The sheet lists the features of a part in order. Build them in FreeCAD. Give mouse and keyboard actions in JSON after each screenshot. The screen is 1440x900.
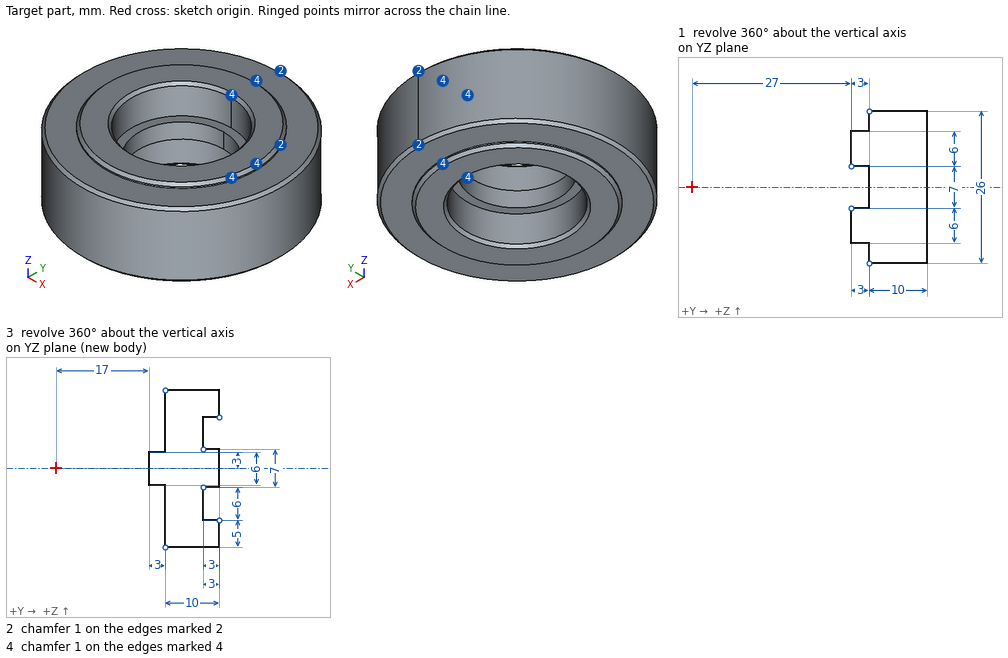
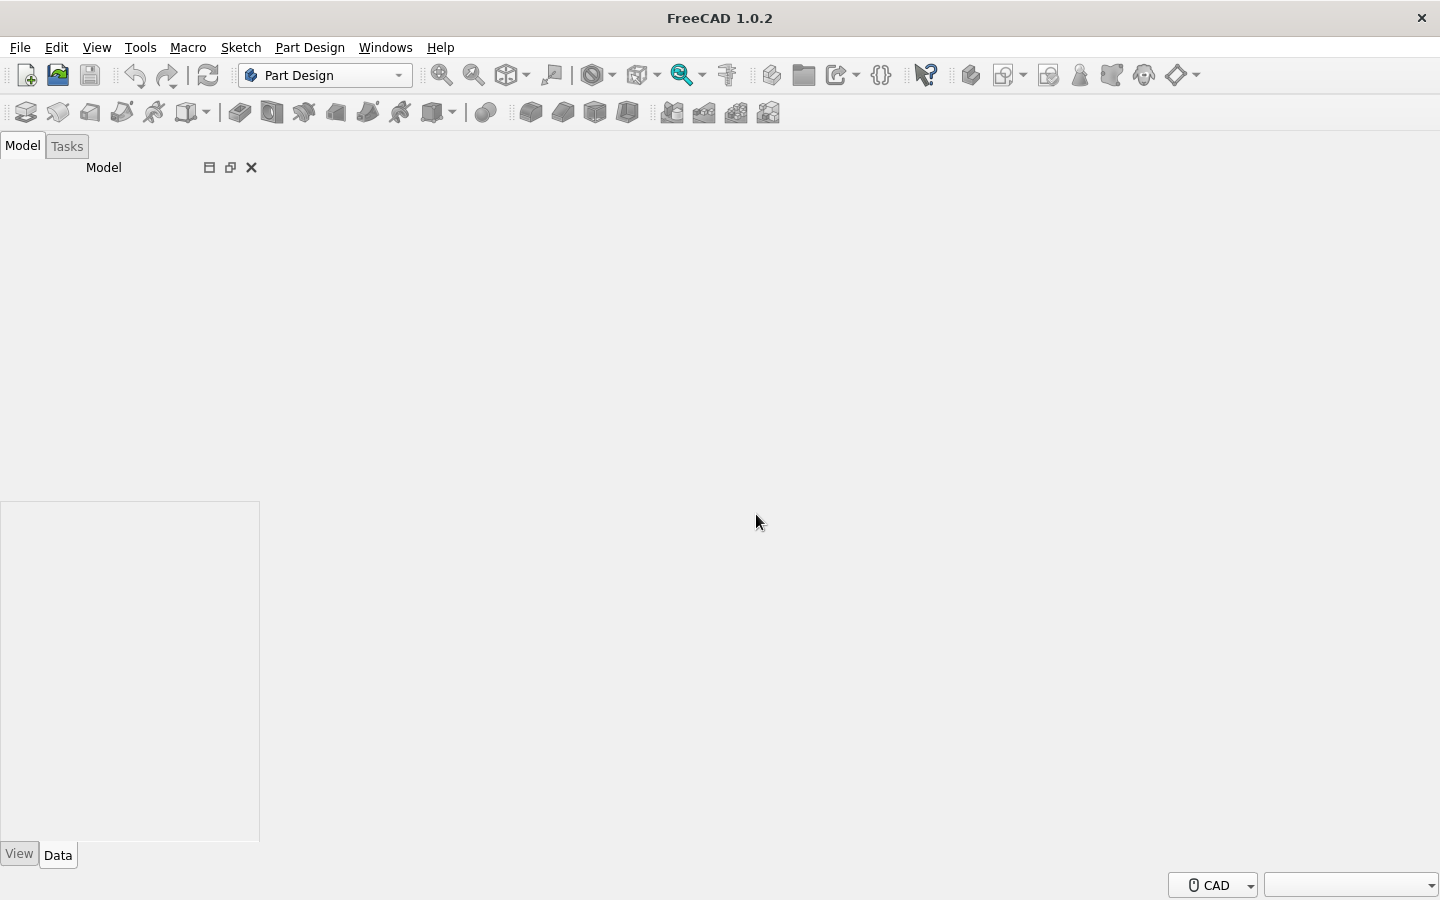
{"action": "left_click", "coordinate": [26, 76]}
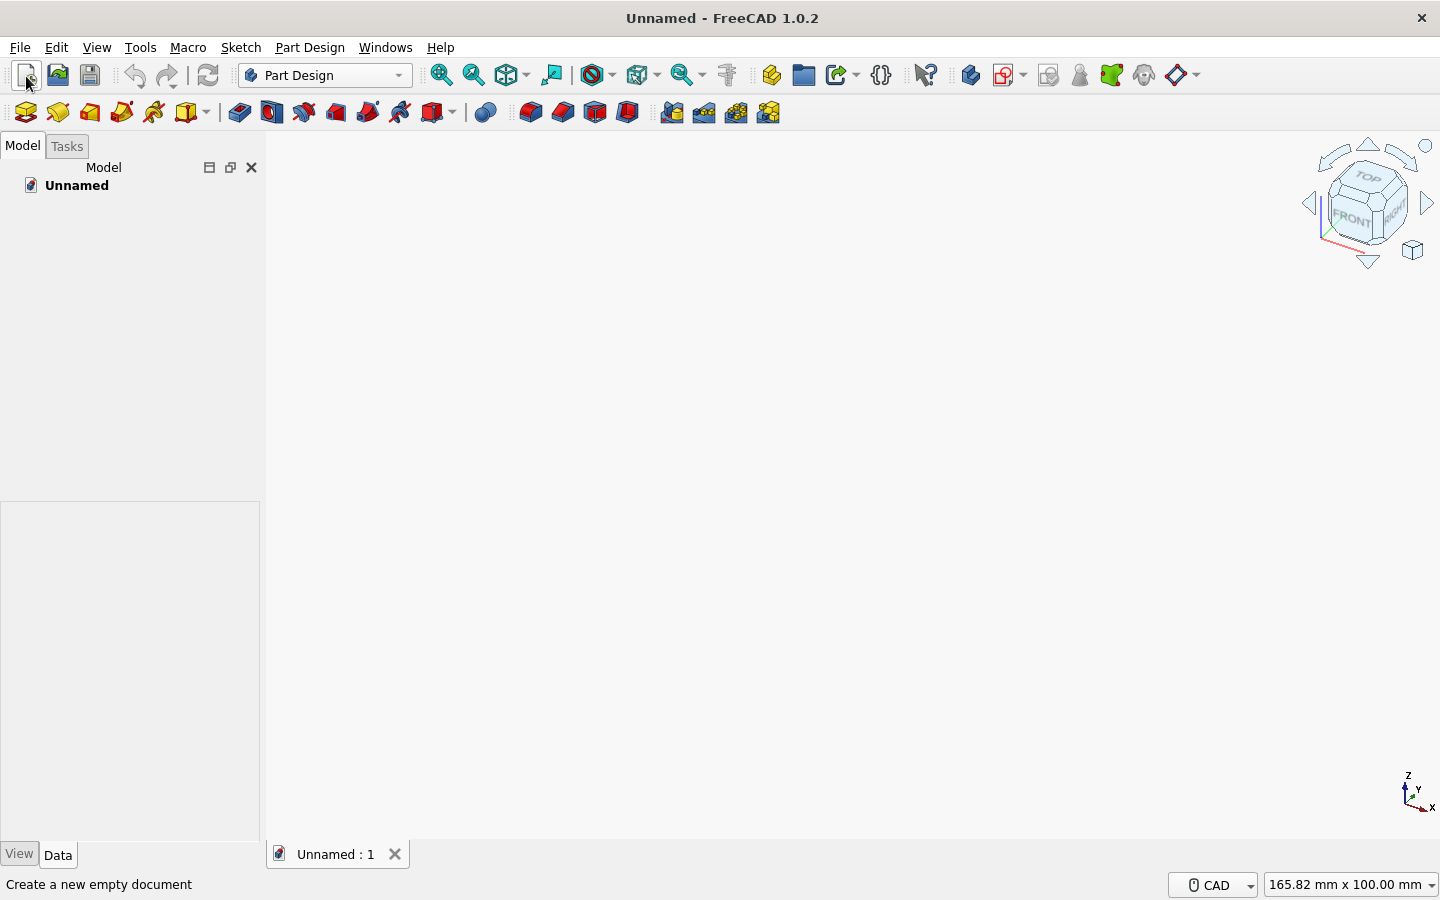
{"action": "left_click", "coordinate": [1004, 76]}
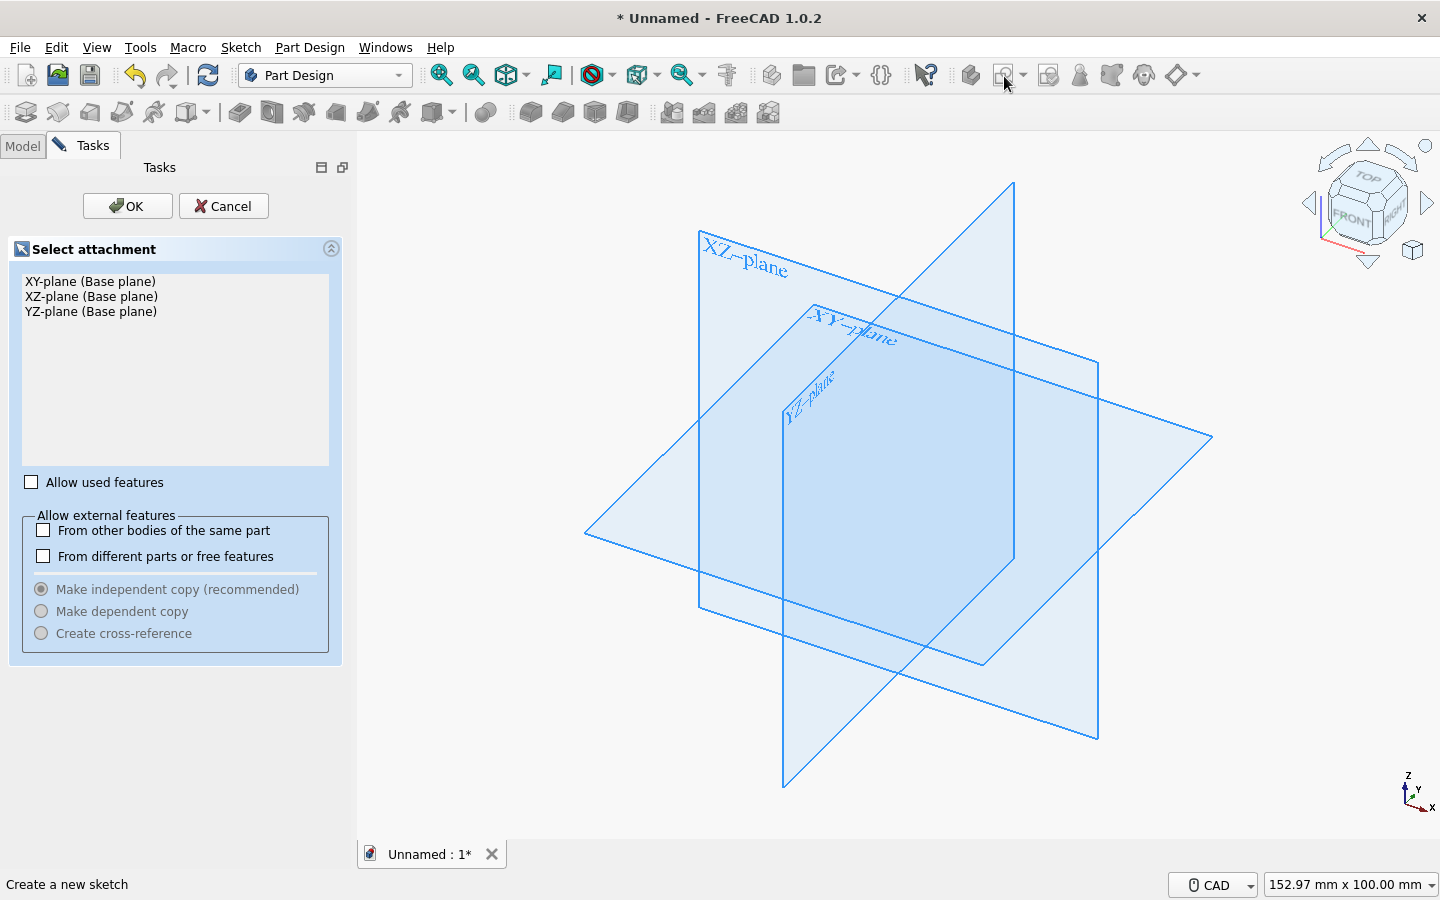
{"action": "left_click", "coordinate": [82, 312]}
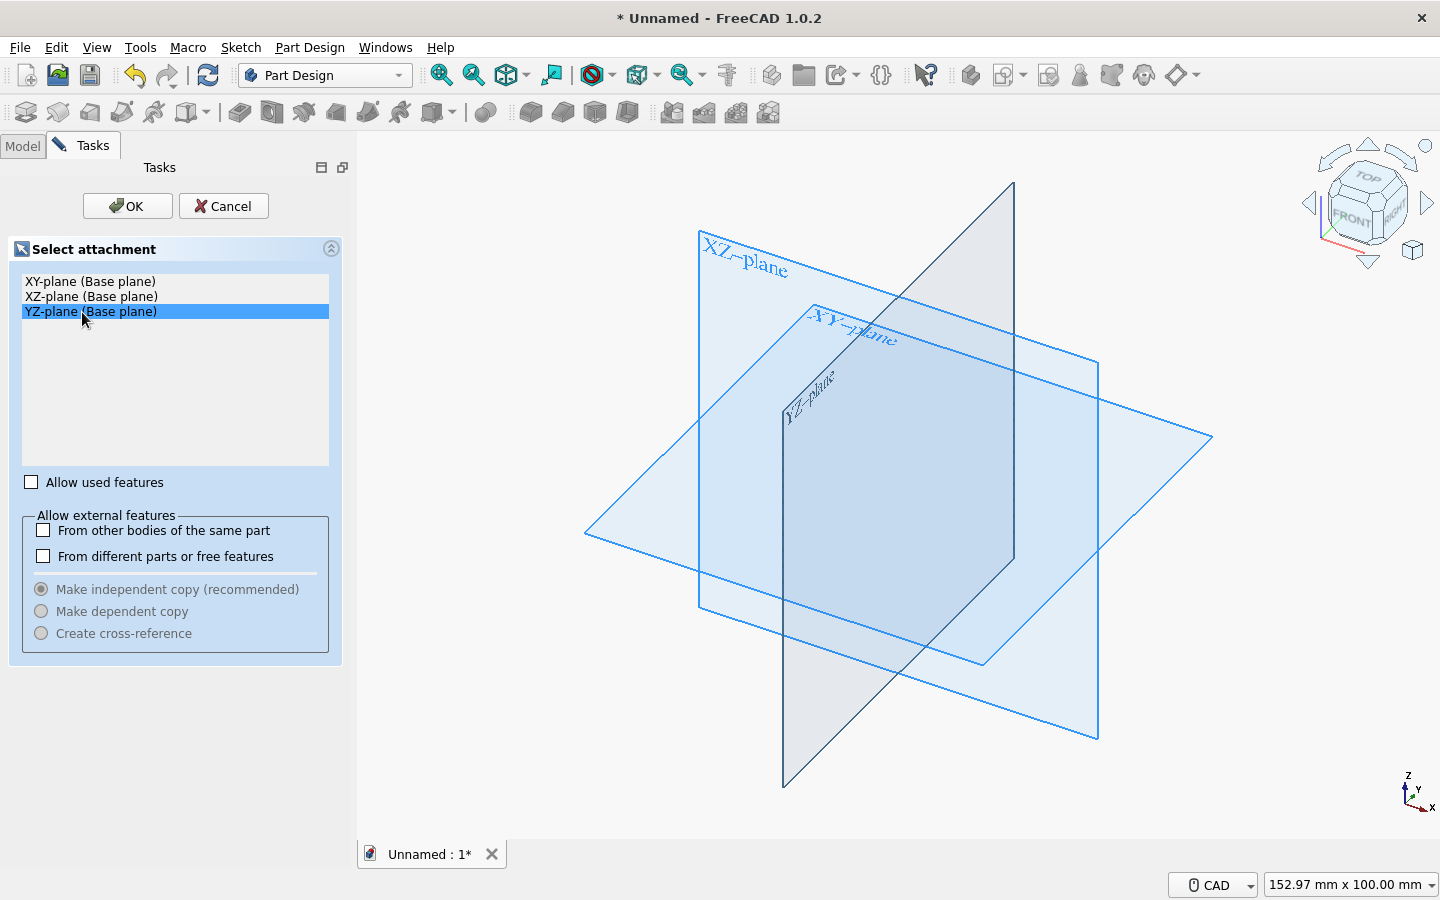
{"action": "left_click", "coordinate": [128, 206]}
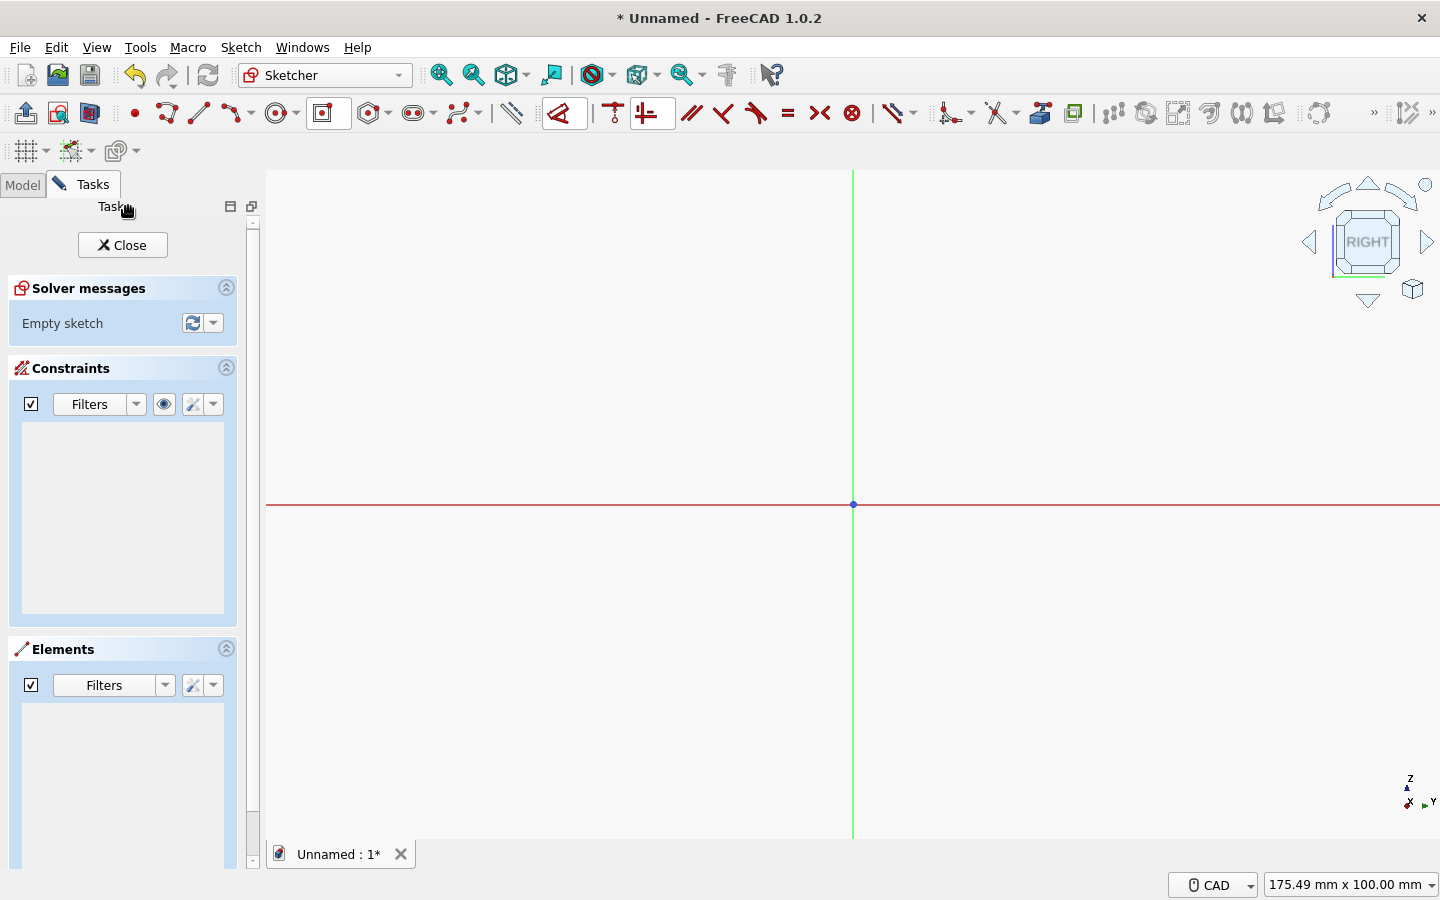
{"action": "scroll", "coordinate": [1105, 504], "scroll_direction": "up", "scroll_amount": 5}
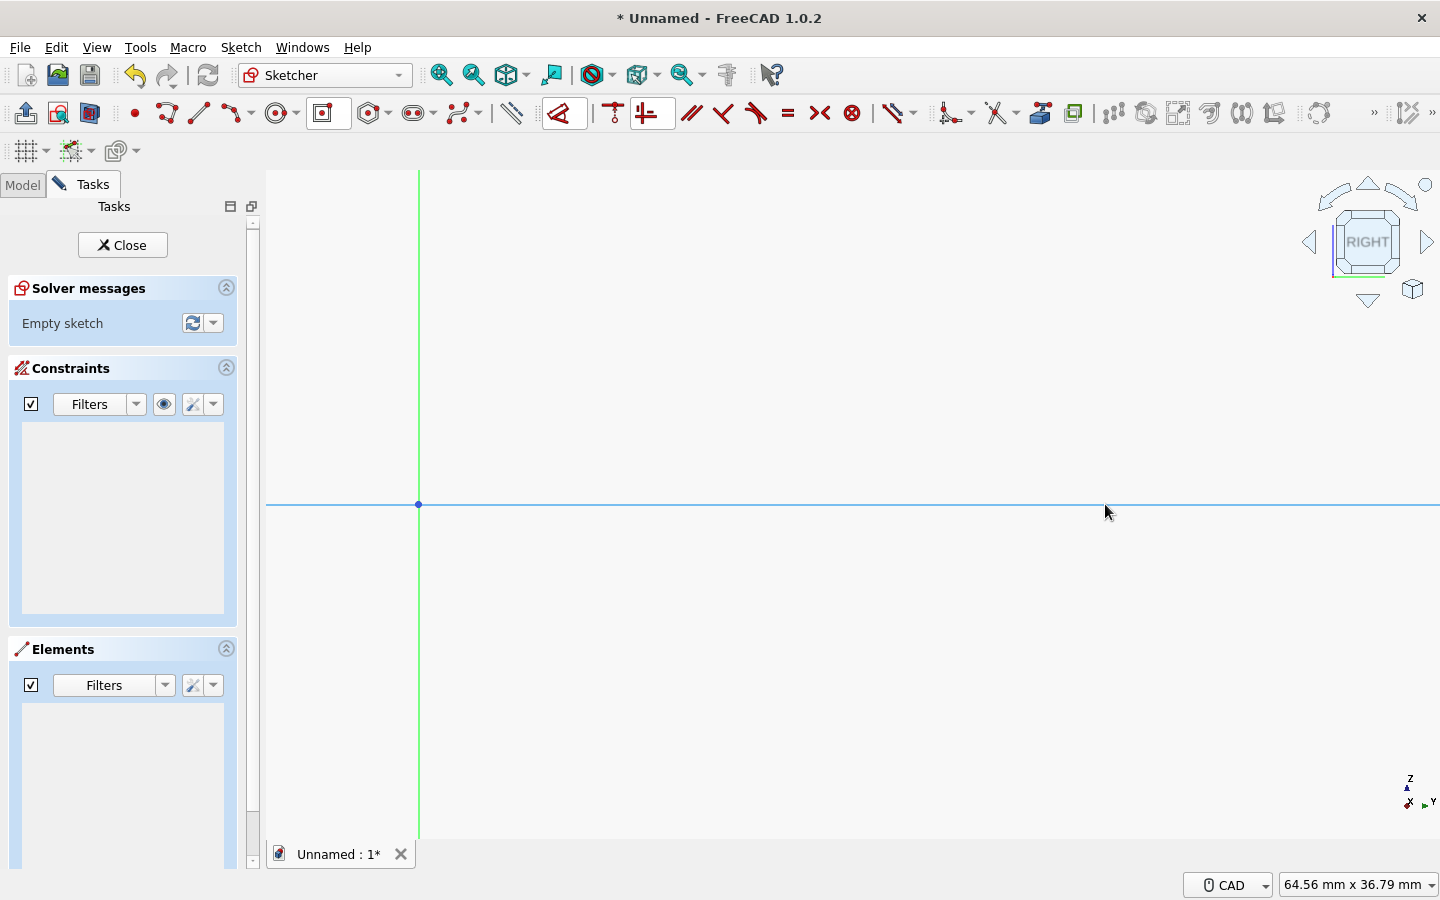
{"action": "left_click", "coordinate": [168, 114]}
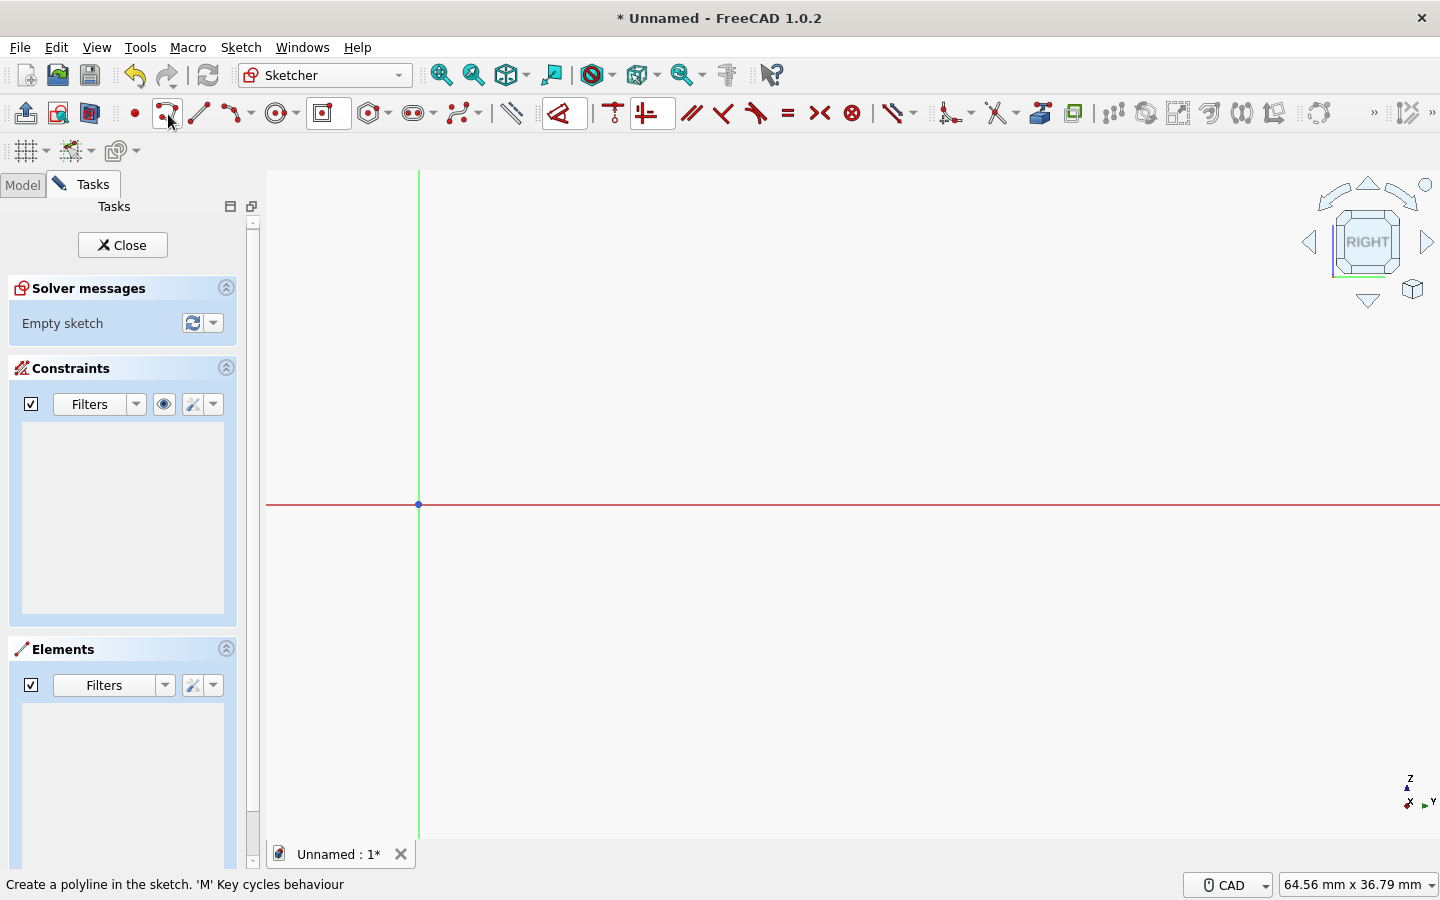
{"action": "left_click", "coordinate": [910, 441]}
{"action": "left_click", "coordinate": [964, 441]}
{"action": "left_click", "coordinate": [964, 568]}
{"action": "left_click", "coordinate": [910, 568]}
{"action": "left_click", "coordinate": [910, 677]}
{"action": "left_click", "coordinate": [964, 677]}
{"action": "left_click", "coordinate": [964, 741]}
{"action": "left_click", "coordinate": [1146, 741]}
{"action": "left_click", "coordinate": [1146, 268]}
{"action": "left_click", "coordinate": [964, 268]}
{"action": "left_click", "coordinate": [964, 332]}
{"action": "left_click", "coordinate": [910, 332]}
{"action": "left_click", "coordinate": [910, 442]}
{"action": "key", "text": "Escape"}
{"action": "key", "text": "Escape"}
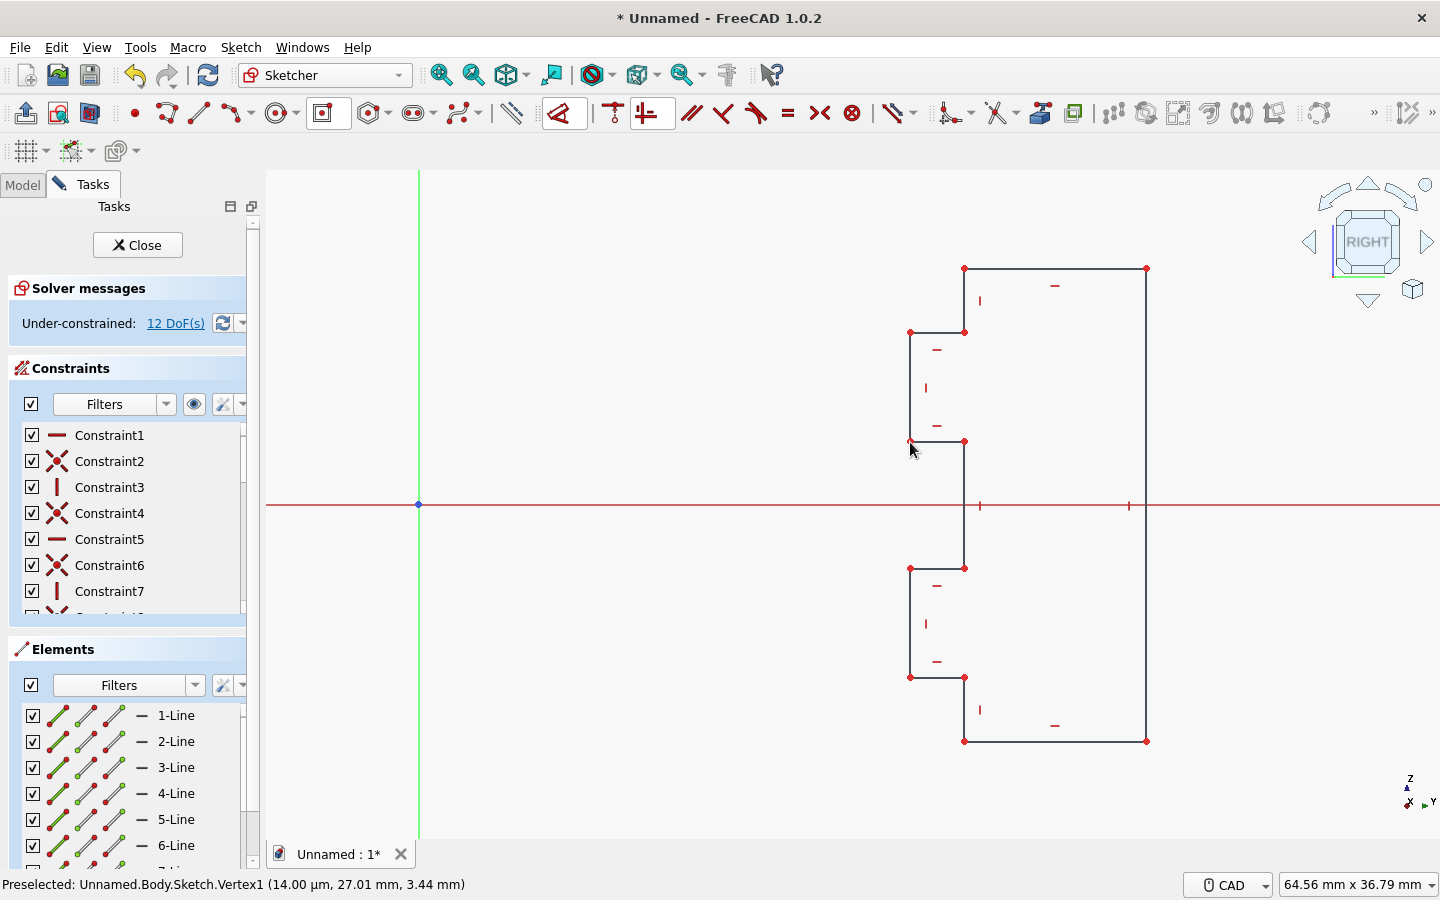
{"action": "left_click", "coordinate": [910, 442]}